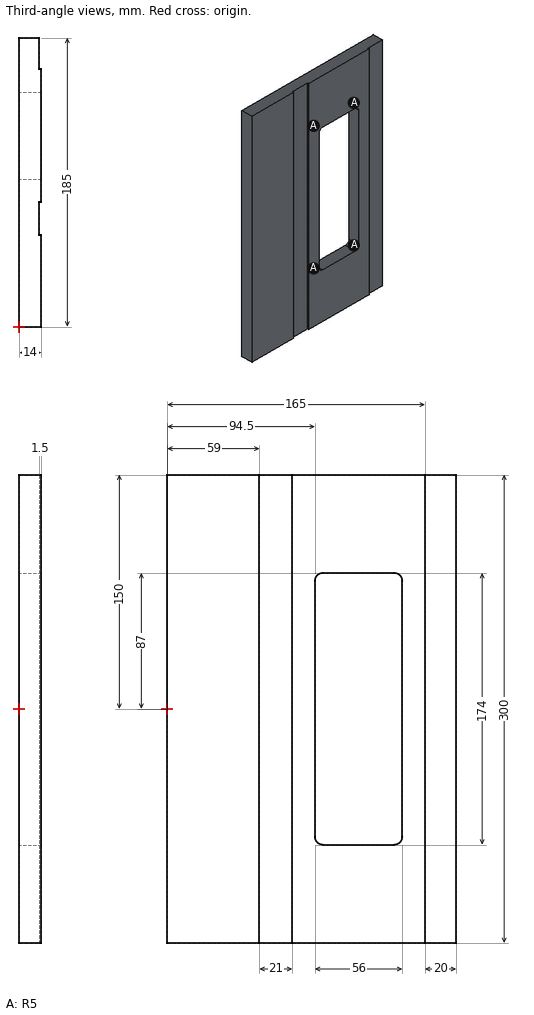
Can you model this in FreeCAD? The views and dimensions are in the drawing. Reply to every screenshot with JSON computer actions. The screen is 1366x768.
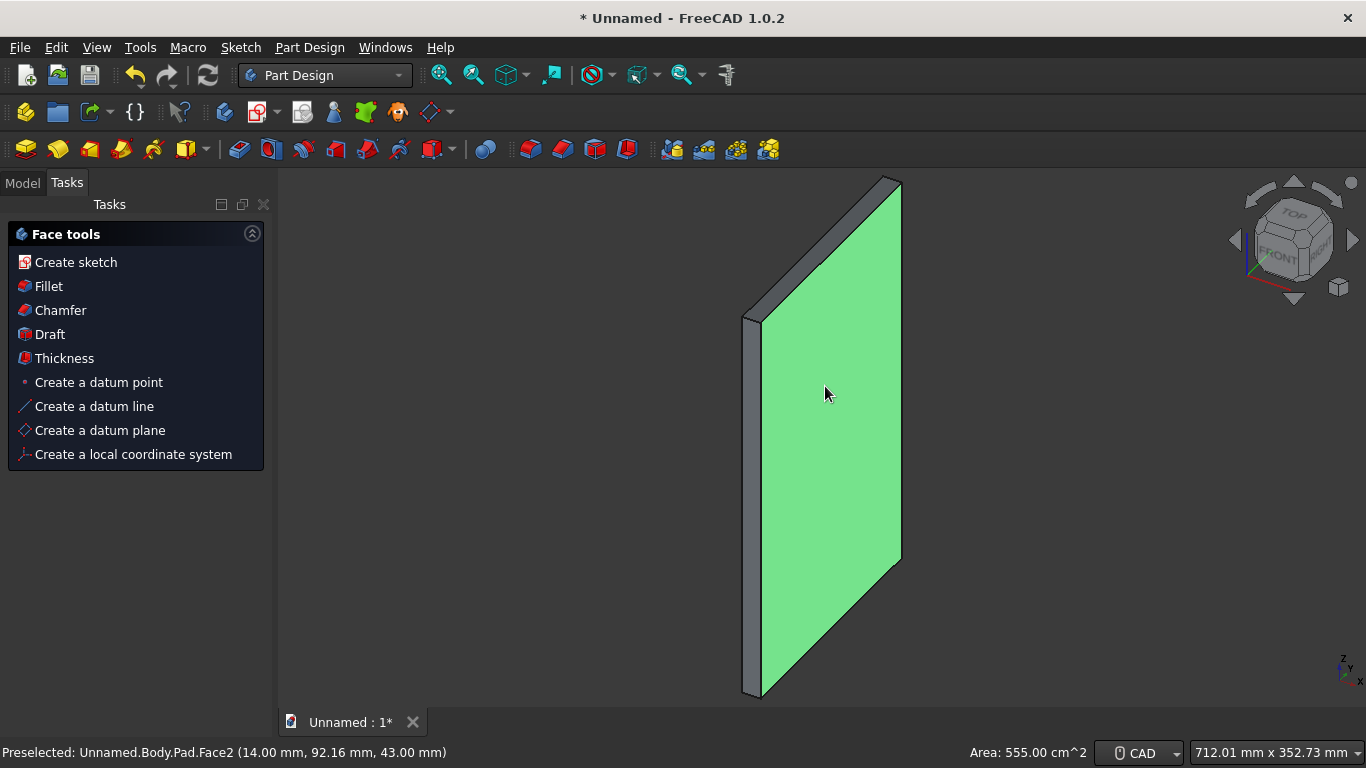
{"action": "left_click", "coordinate": [258, 112]}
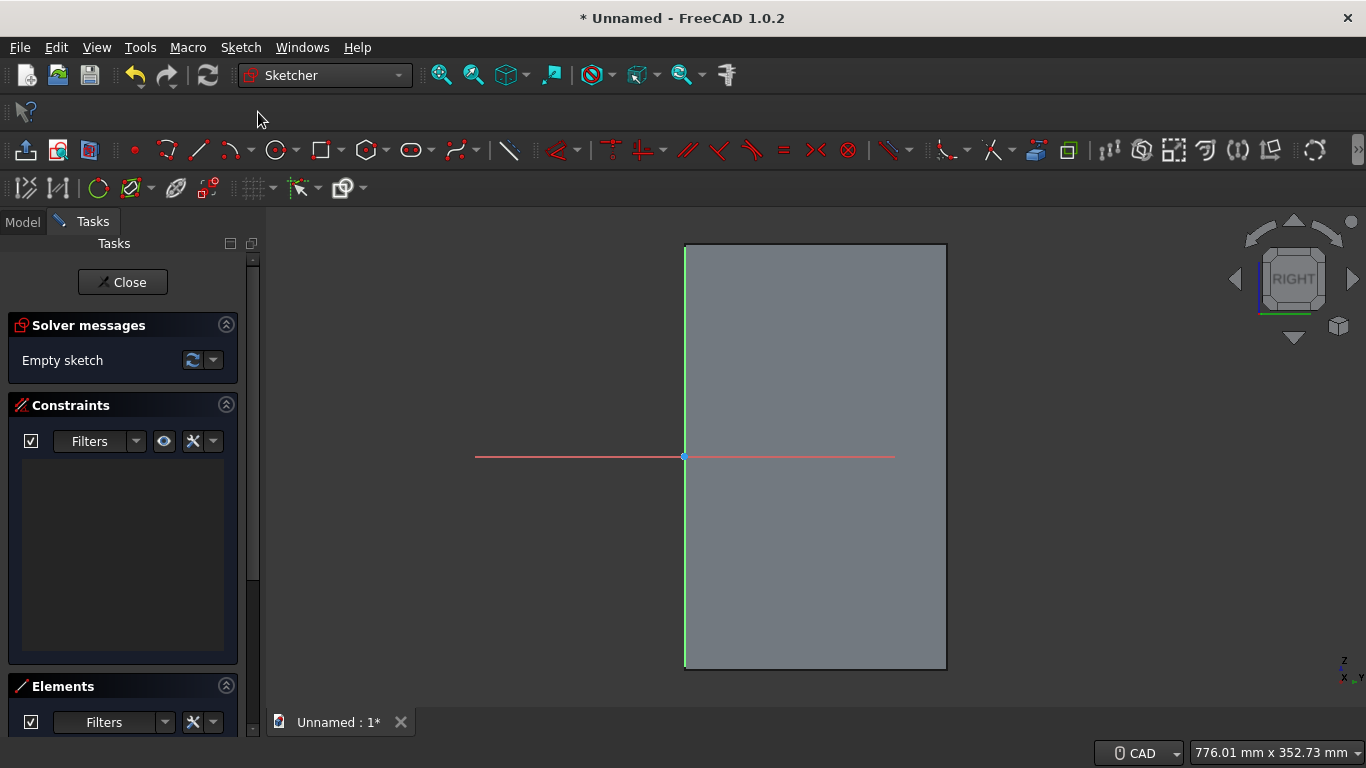
{"action": "scroll", "coordinate": [608, 457], "scroll_direction": "down", "scroll_amount": 2}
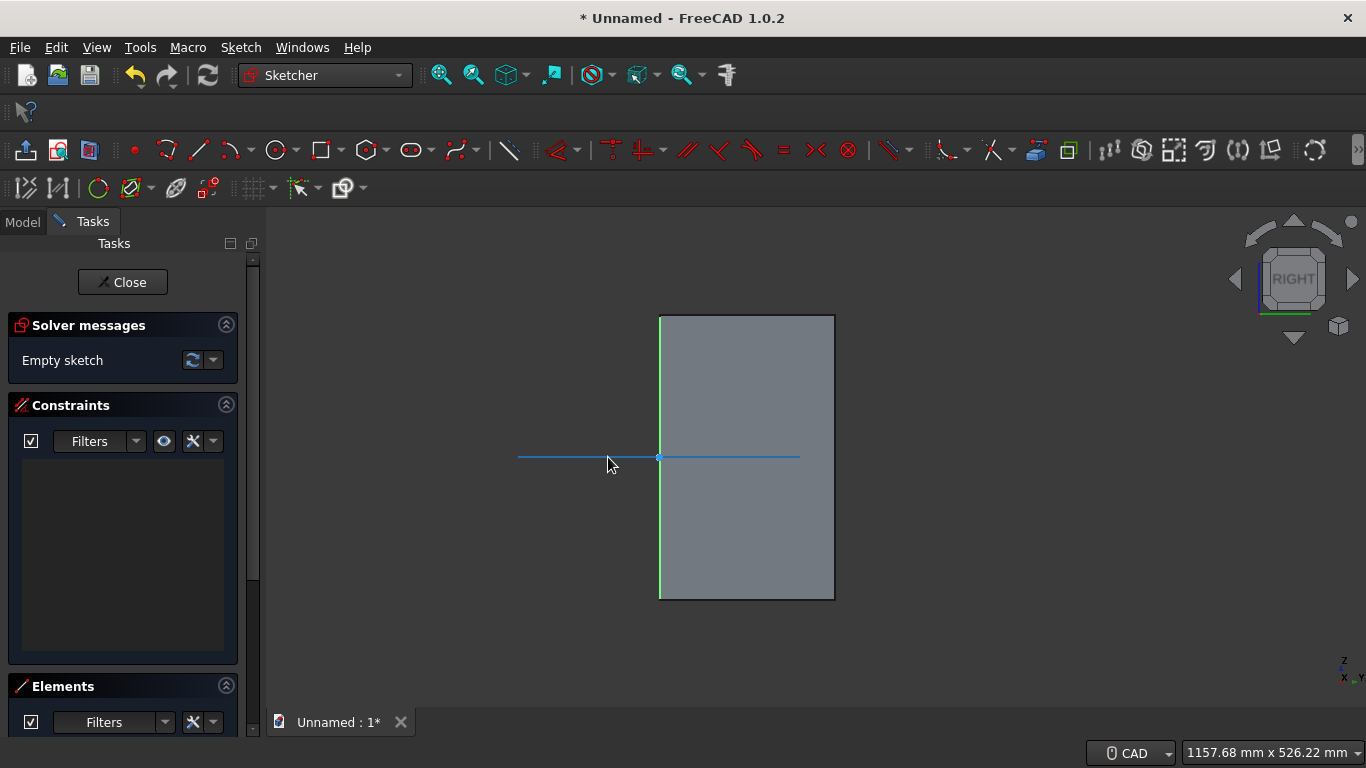
{"action": "left_click", "coordinate": [322, 150]}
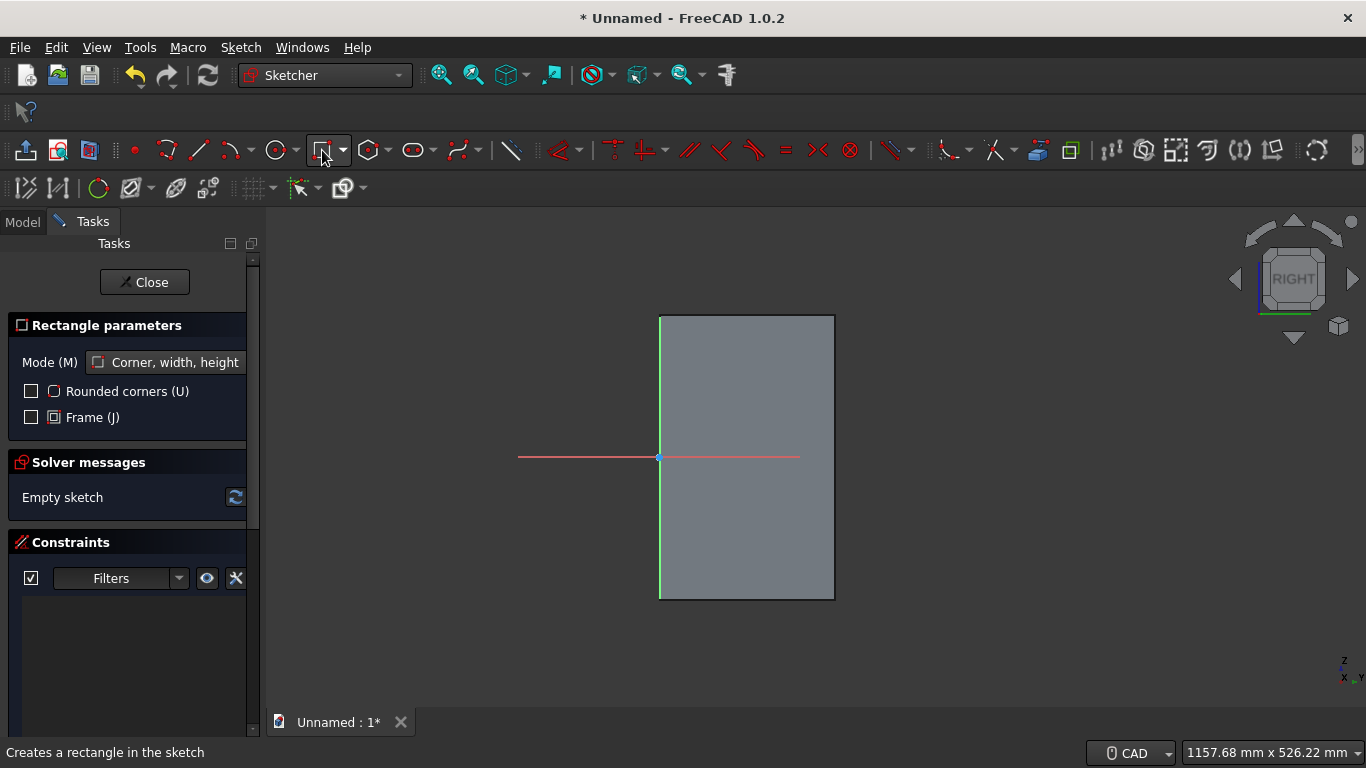
{"action": "left_click", "coordinate": [816, 315]}
{"action": "left_click", "coordinate": [835, 600]}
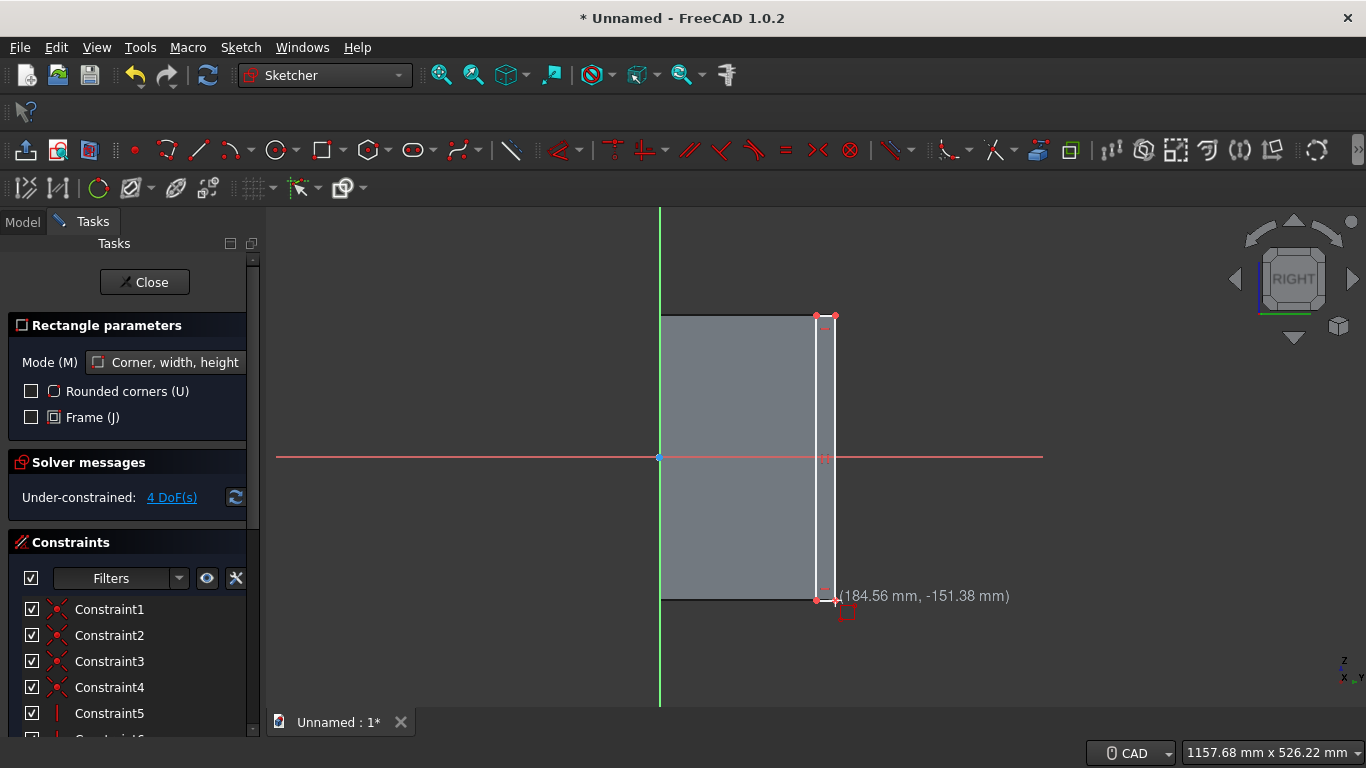
{"action": "left_click", "coordinate": [716, 315]}
{"action": "left_click", "coordinate": [736, 600]}
{"action": "key", "text": "Escape"}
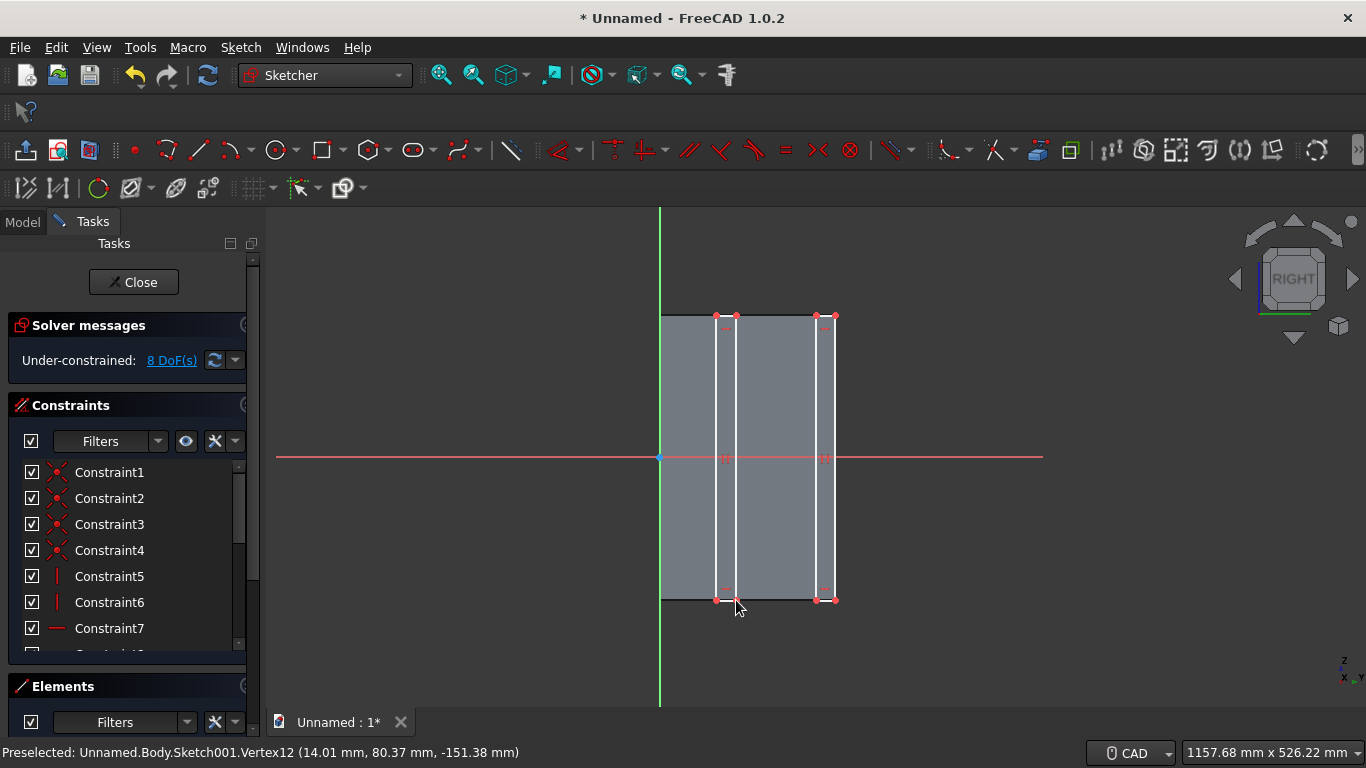
{"action": "left_click", "coordinate": [558, 150]}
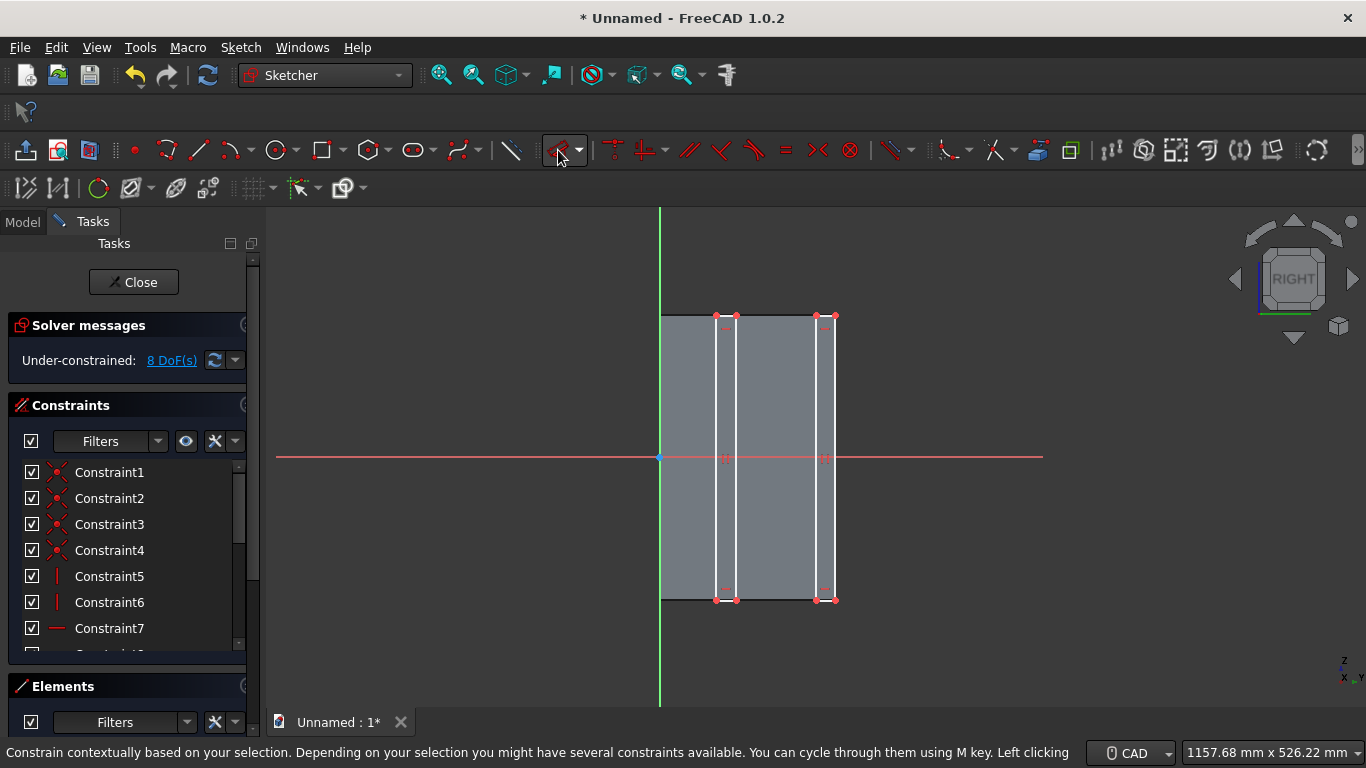
{"action": "scroll", "coordinate": [825, 601], "scroll_direction": "up", "scroll_amount": 4}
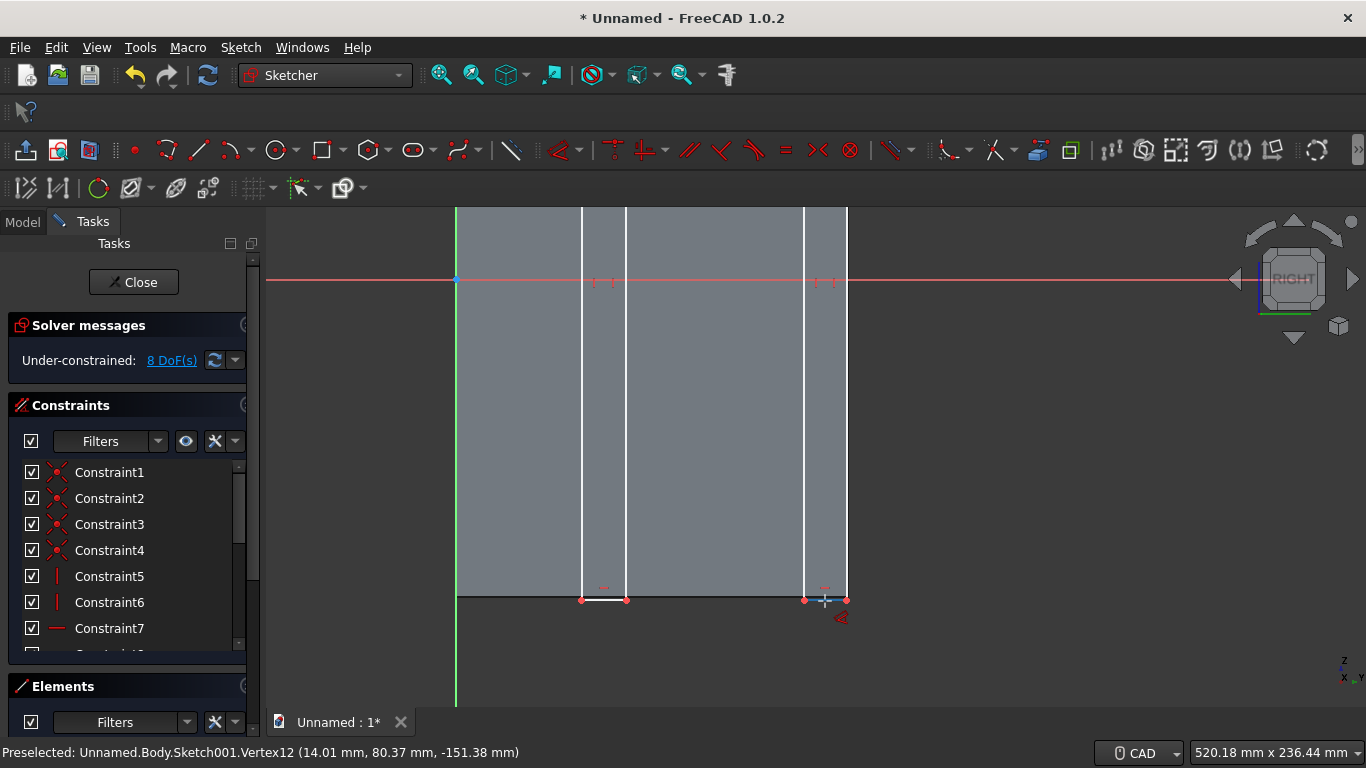
{"action": "left_click", "coordinate": [825, 600]}
{"action": "left_click", "coordinate": [825, 634]}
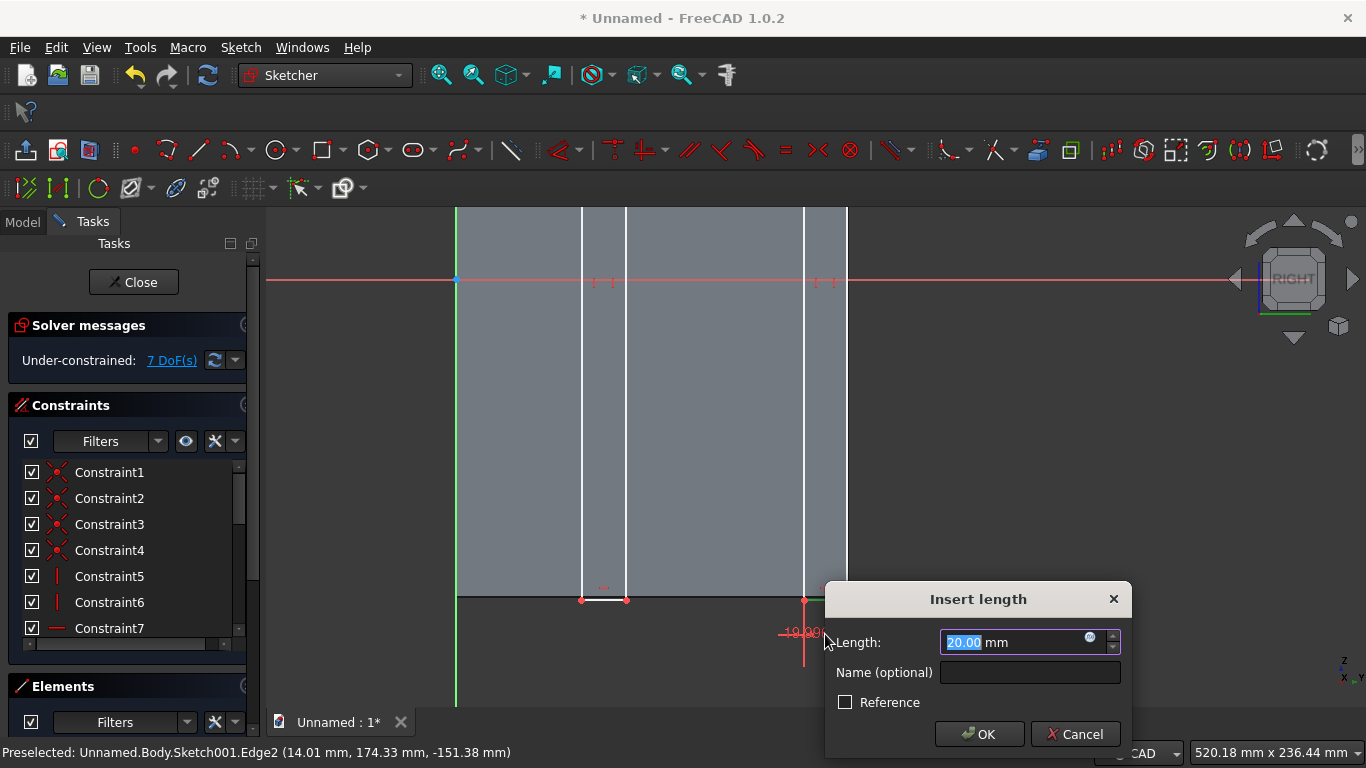
{"action": "type", "text": "20"}
{"action": "key", "text": "Return"}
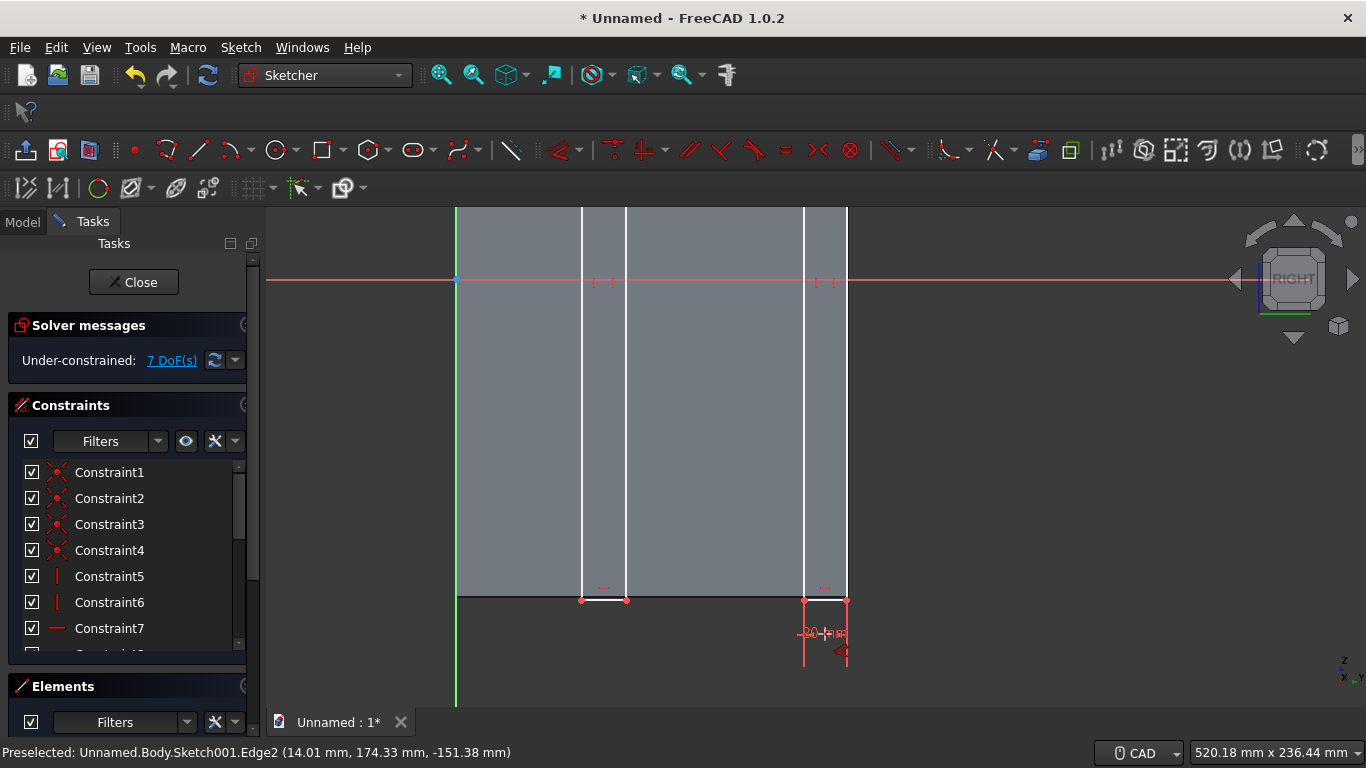
{"action": "left_click", "coordinate": [595, 600]}
{"action": "left_click", "coordinate": [604, 634]}